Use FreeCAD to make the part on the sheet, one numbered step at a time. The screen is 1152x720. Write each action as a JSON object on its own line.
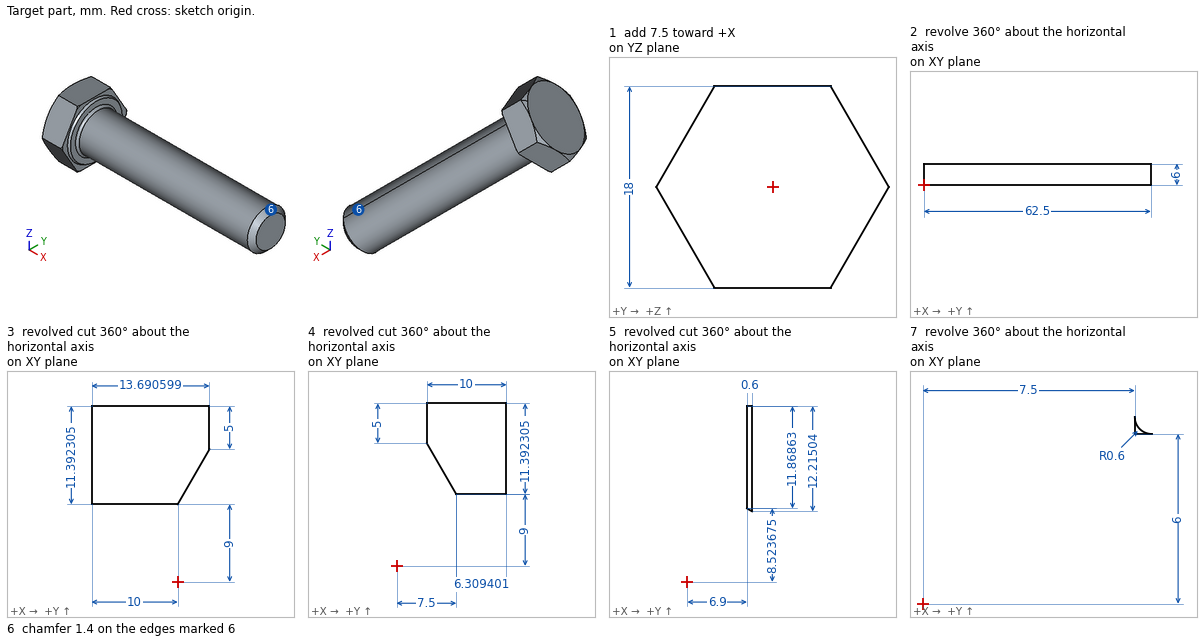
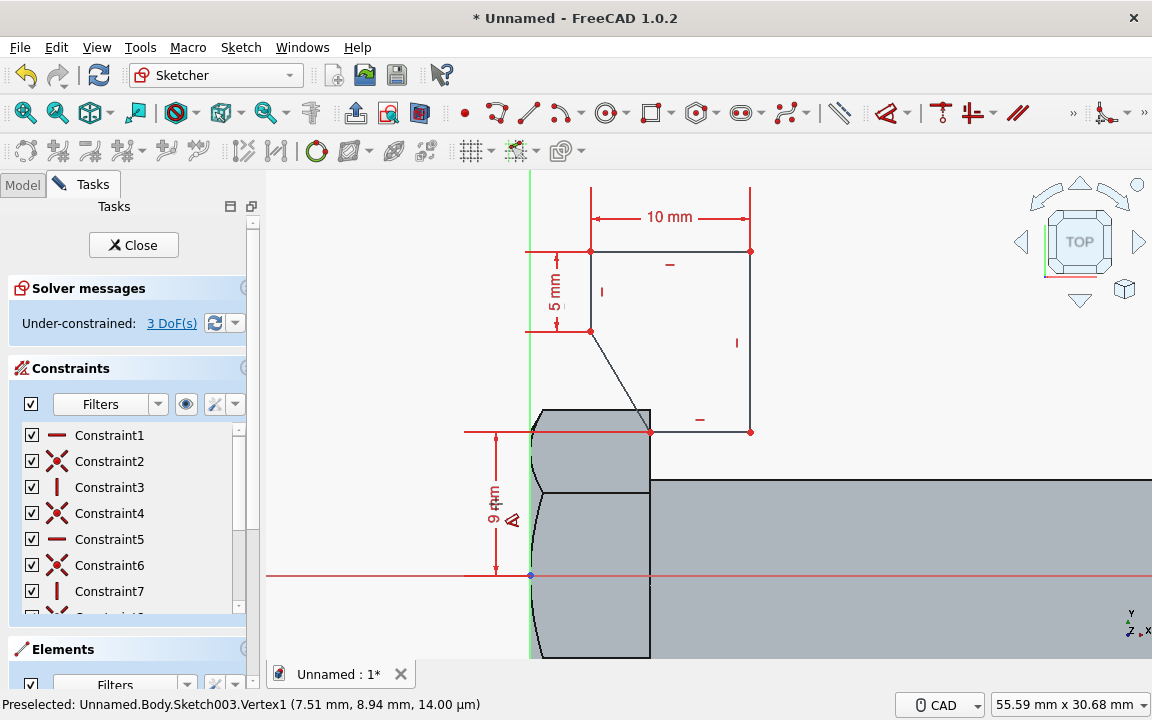
{"action": "left_click", "coordinate": [650, 432]}
{"action": "left_click", "coordinate": [590, 610]}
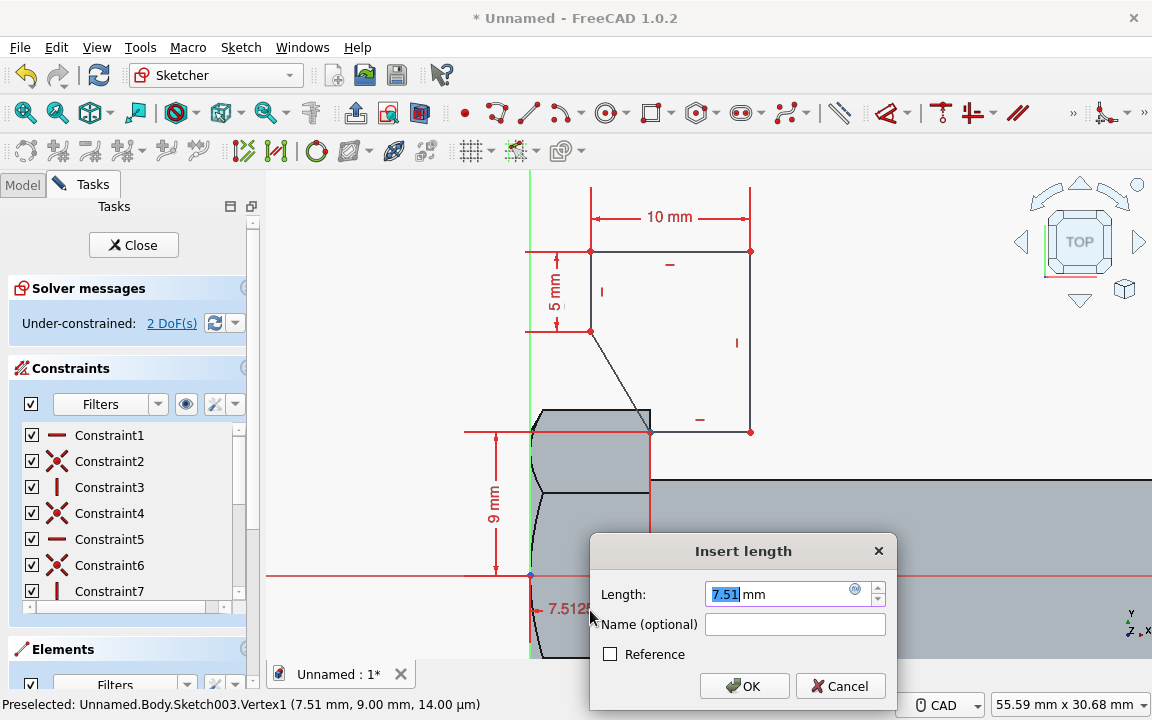
{"action": "type", "text": "7.5"}
{"action": "key", "text": "Return"}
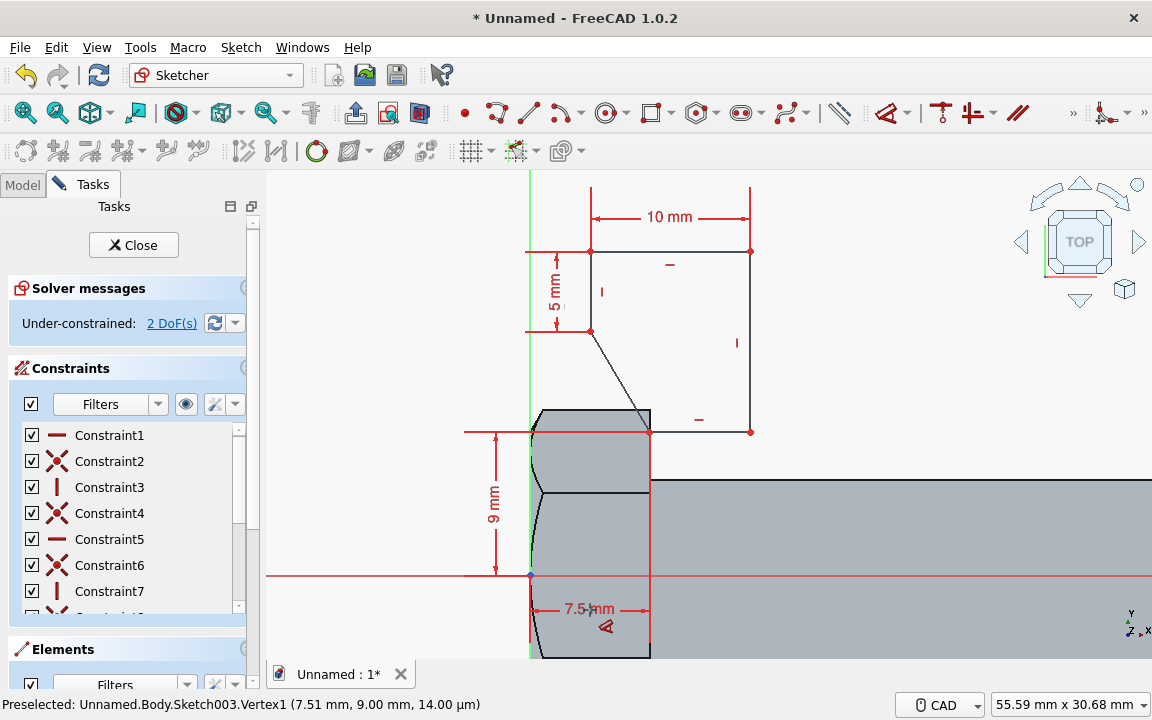
{"action": "left_click", "coordinate": [680, 432]}
{"action": "left_click", "coordinate": [700, 466]}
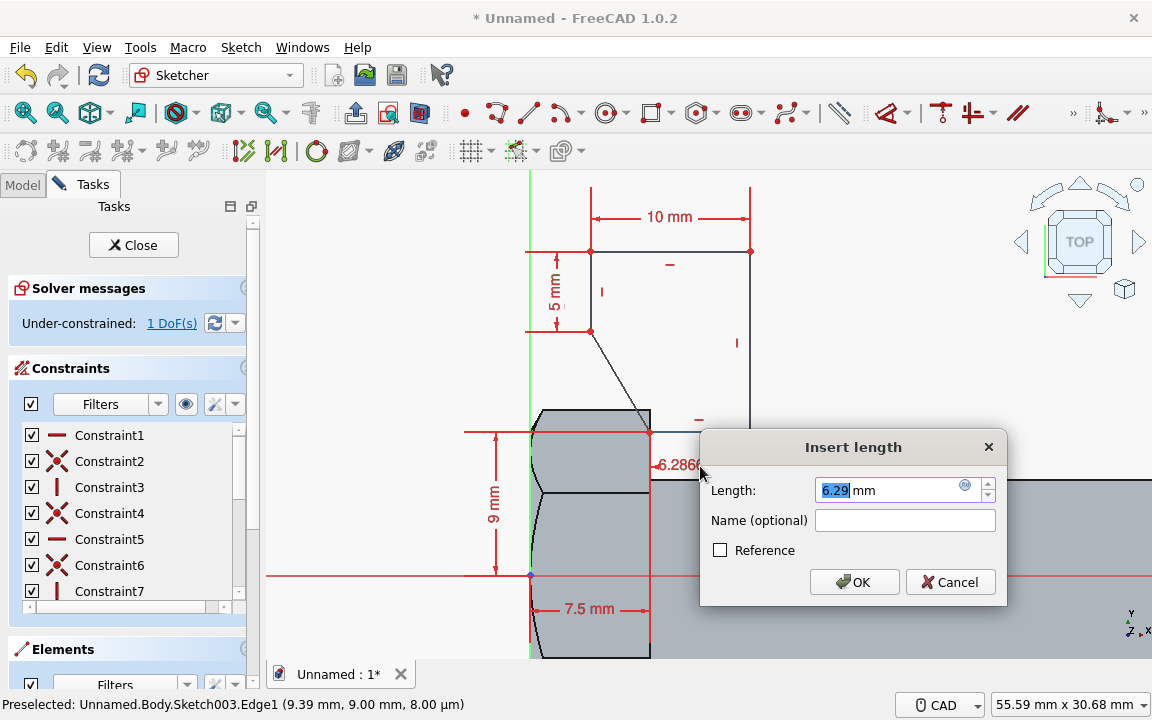
{"action": "type", "text": "6.309401"}
{"action": "key", "text": "Return"}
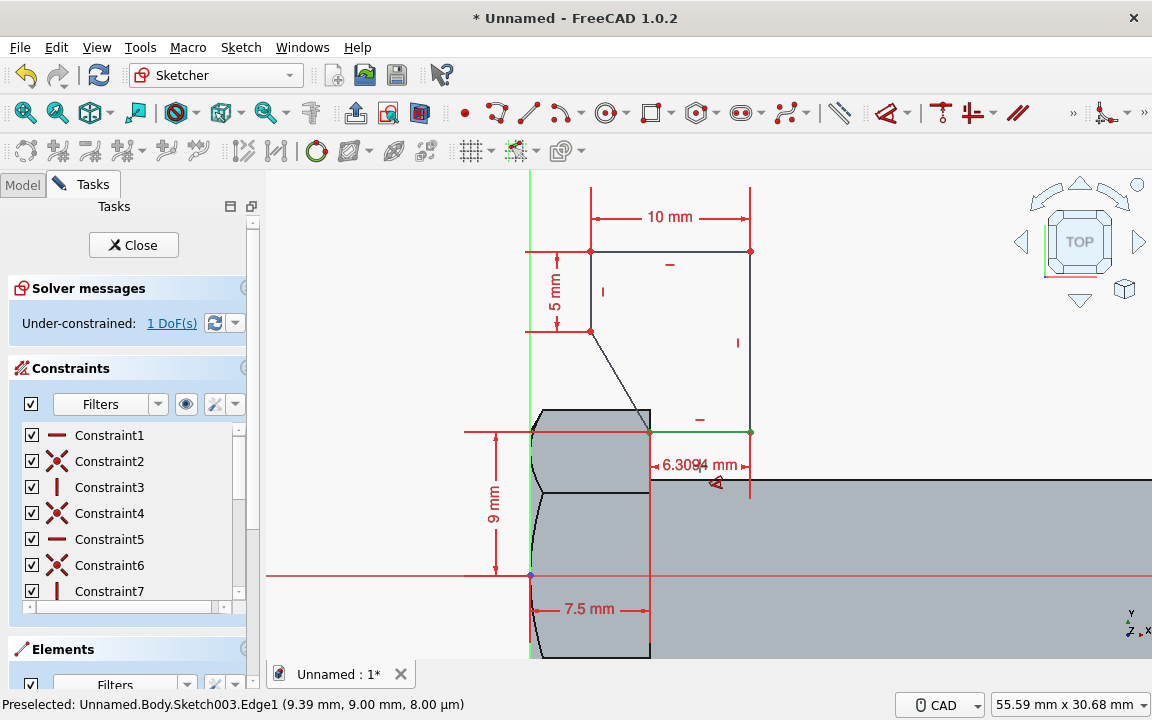
{"action": "left_click", "coordinate": [750, 378]}
{"action": "left_click", "coordinate": [784, 342]}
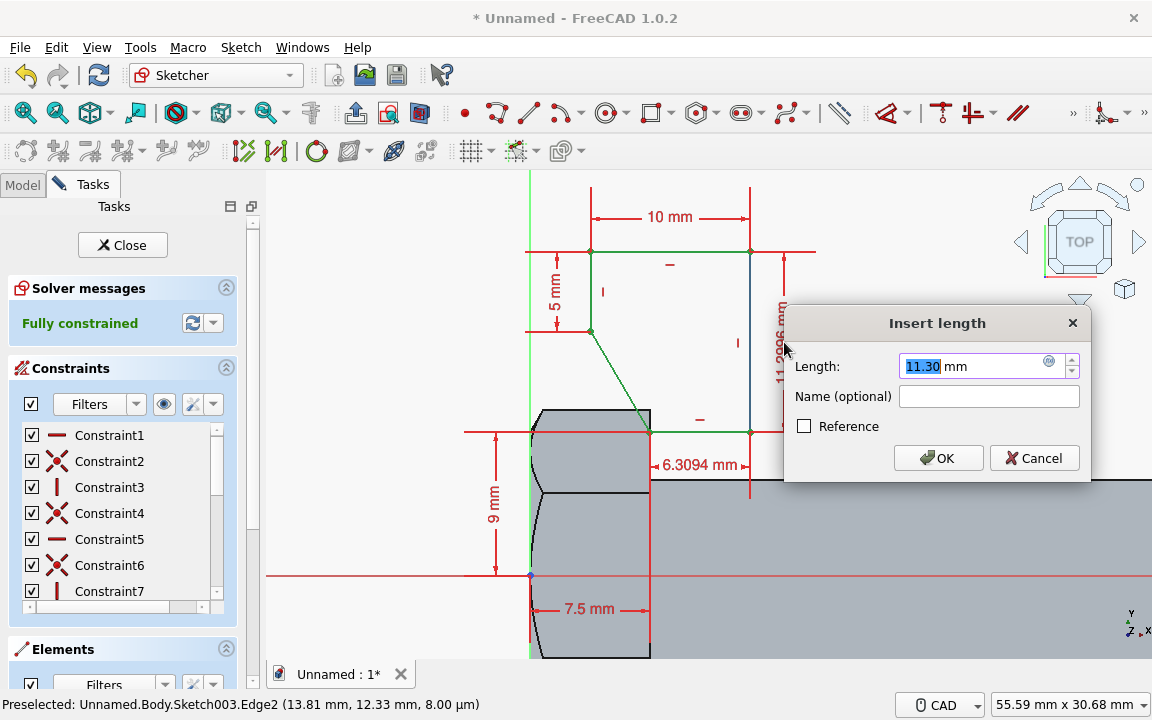
{"action": "type", "text": "11.392305"}
{"action": "key", "text": "Return"}
{"action": "key", "text": "Escape"}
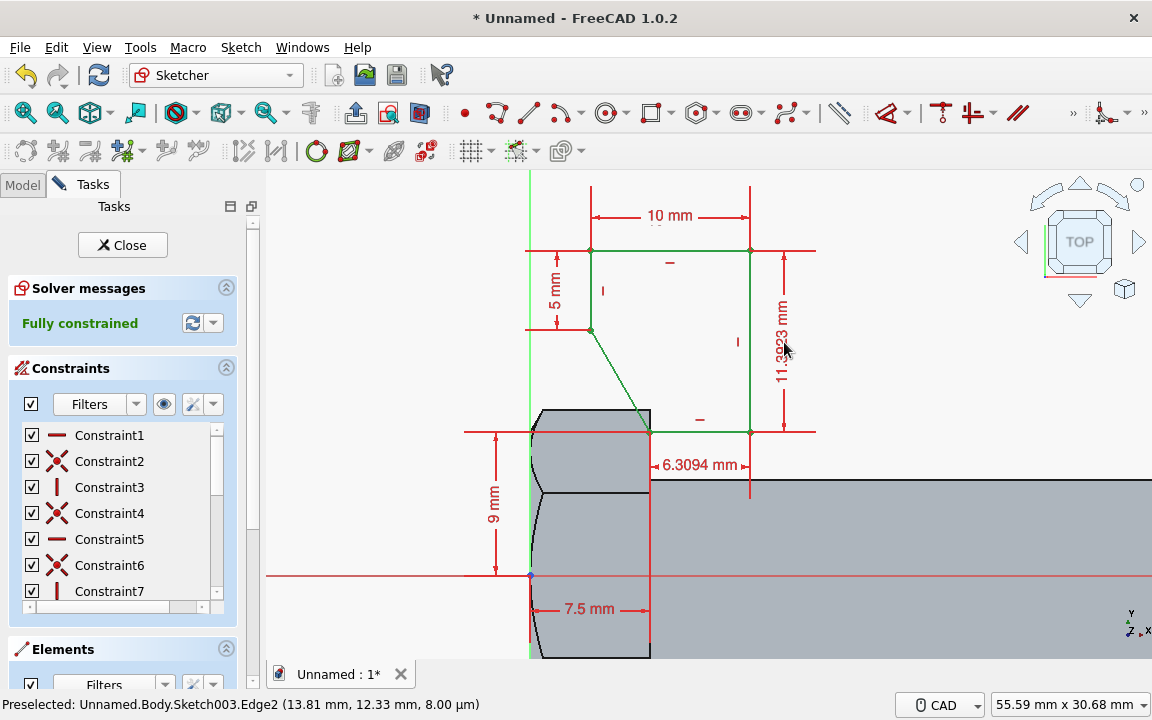
{"action": "left_click", "coordinate": [123, 245]}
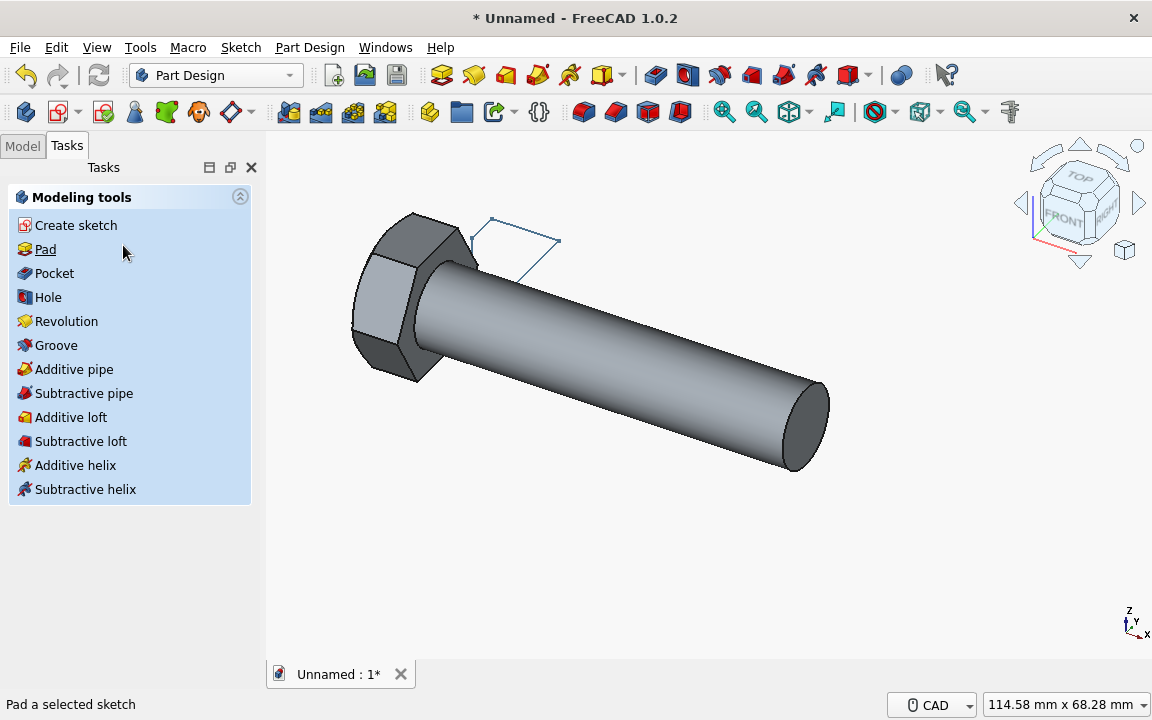
{"action": "left_click", "coordinate": [720, 76]}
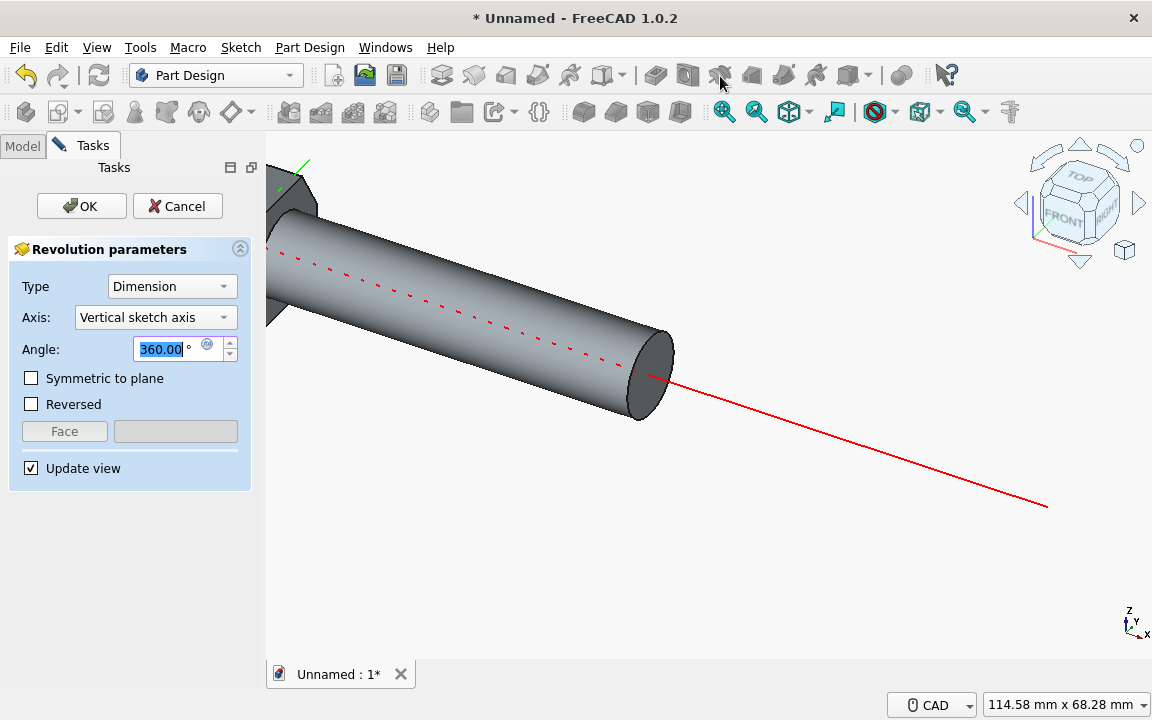
{"action": "left_click", "coordinate": [156, 318]}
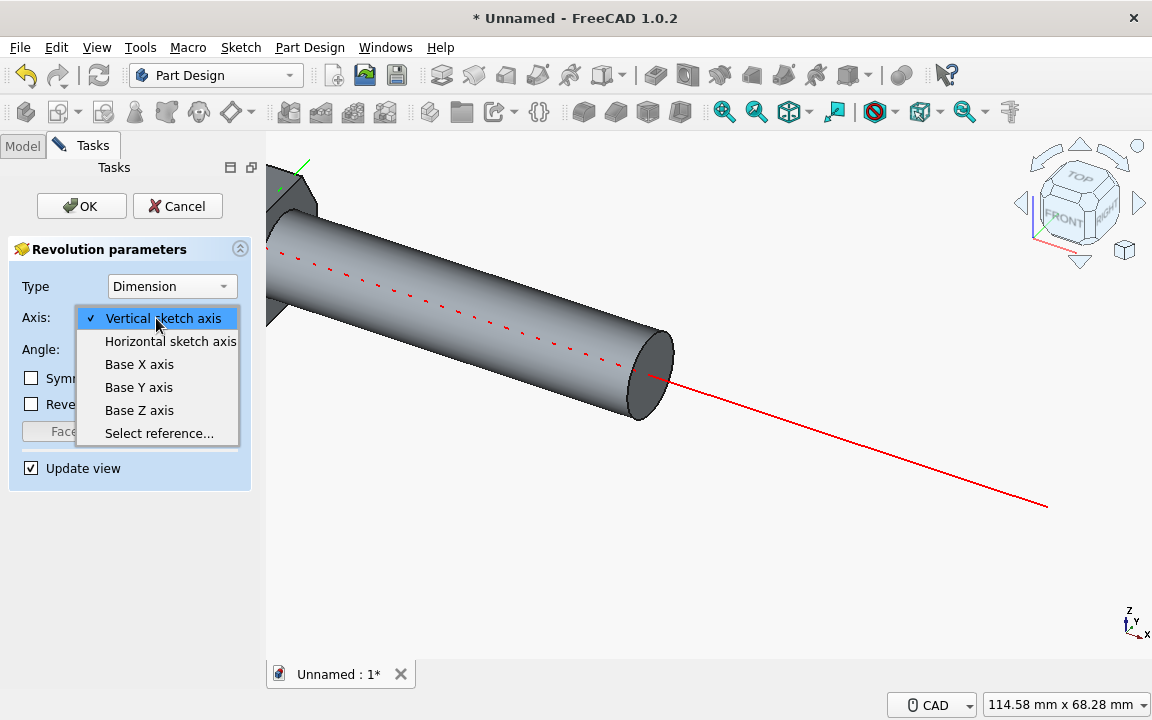
{"action": "left_click", "coordinate": [156, 342]}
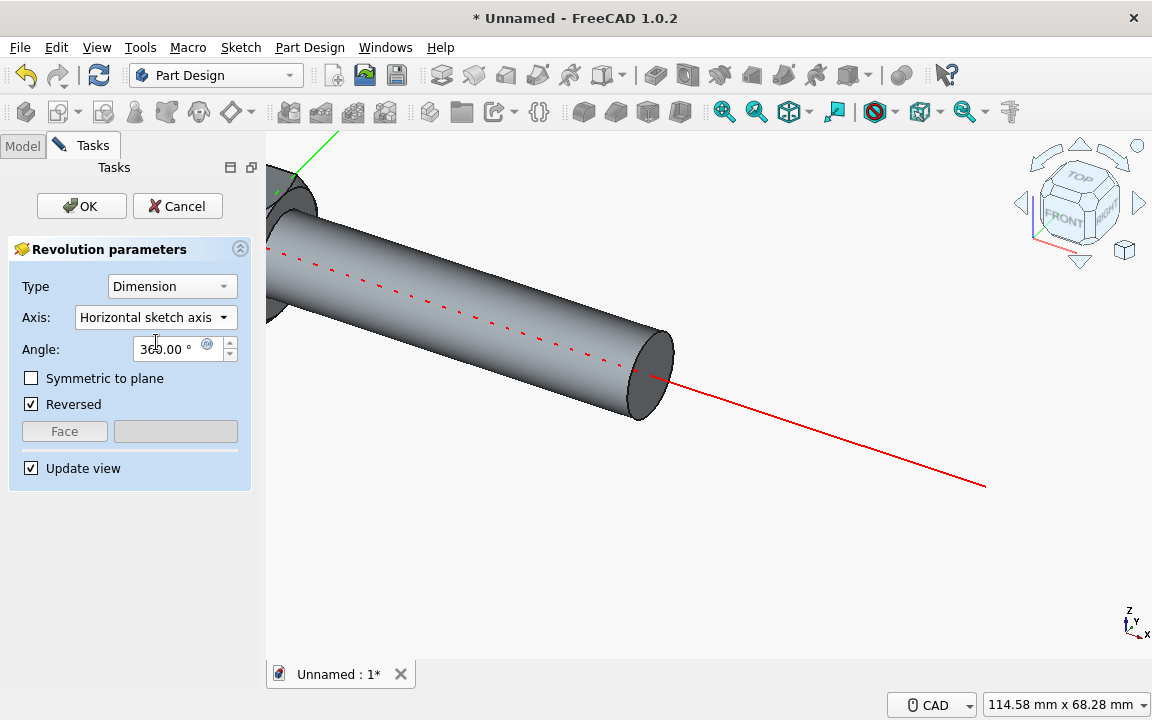
{"action": "left_click", "coordinate": [82, 206]}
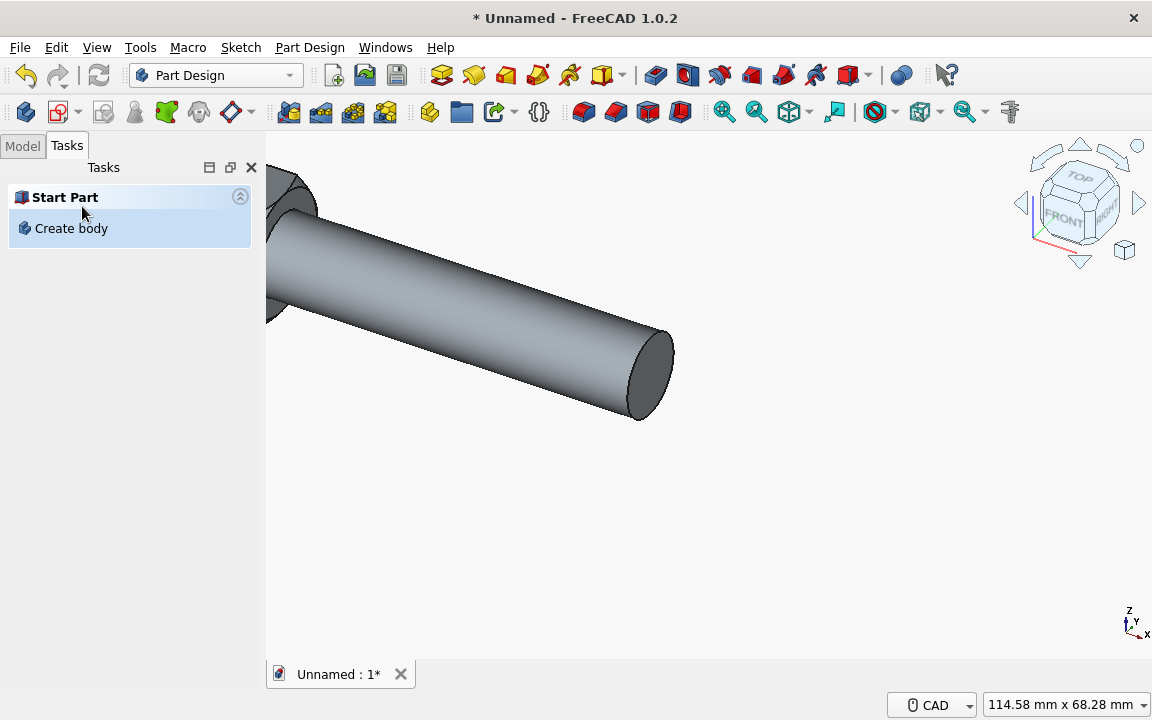
{"action": "left_click", "coordinate": [726, 112]}